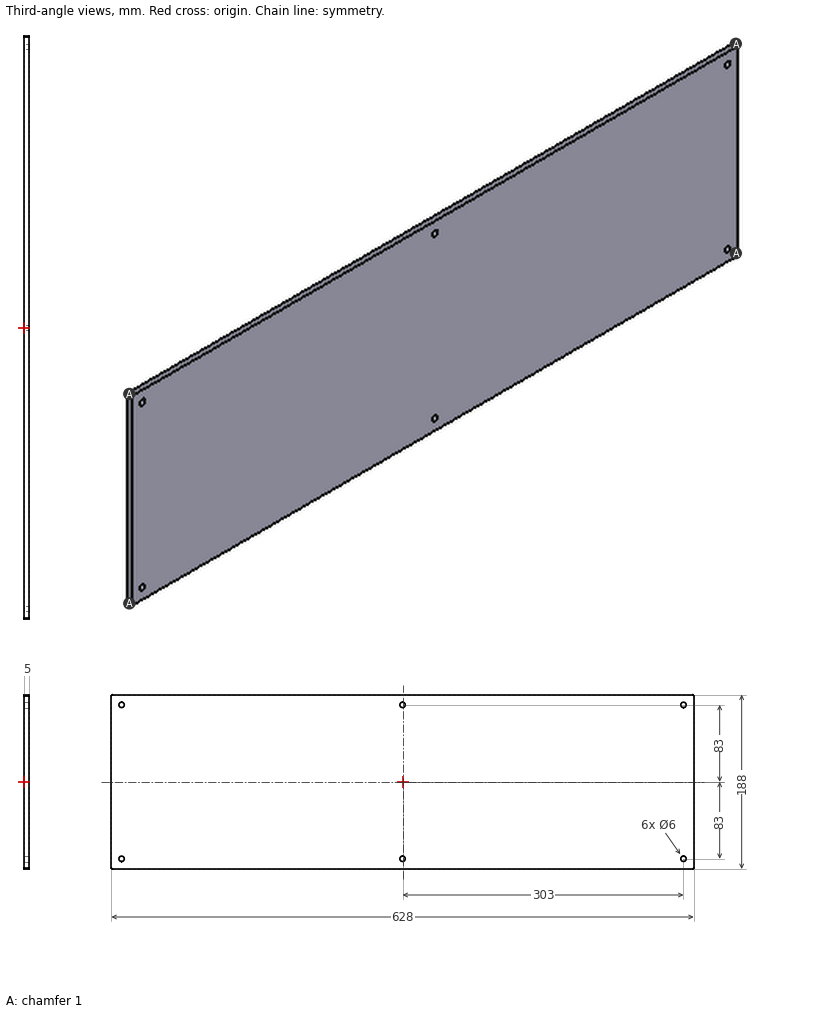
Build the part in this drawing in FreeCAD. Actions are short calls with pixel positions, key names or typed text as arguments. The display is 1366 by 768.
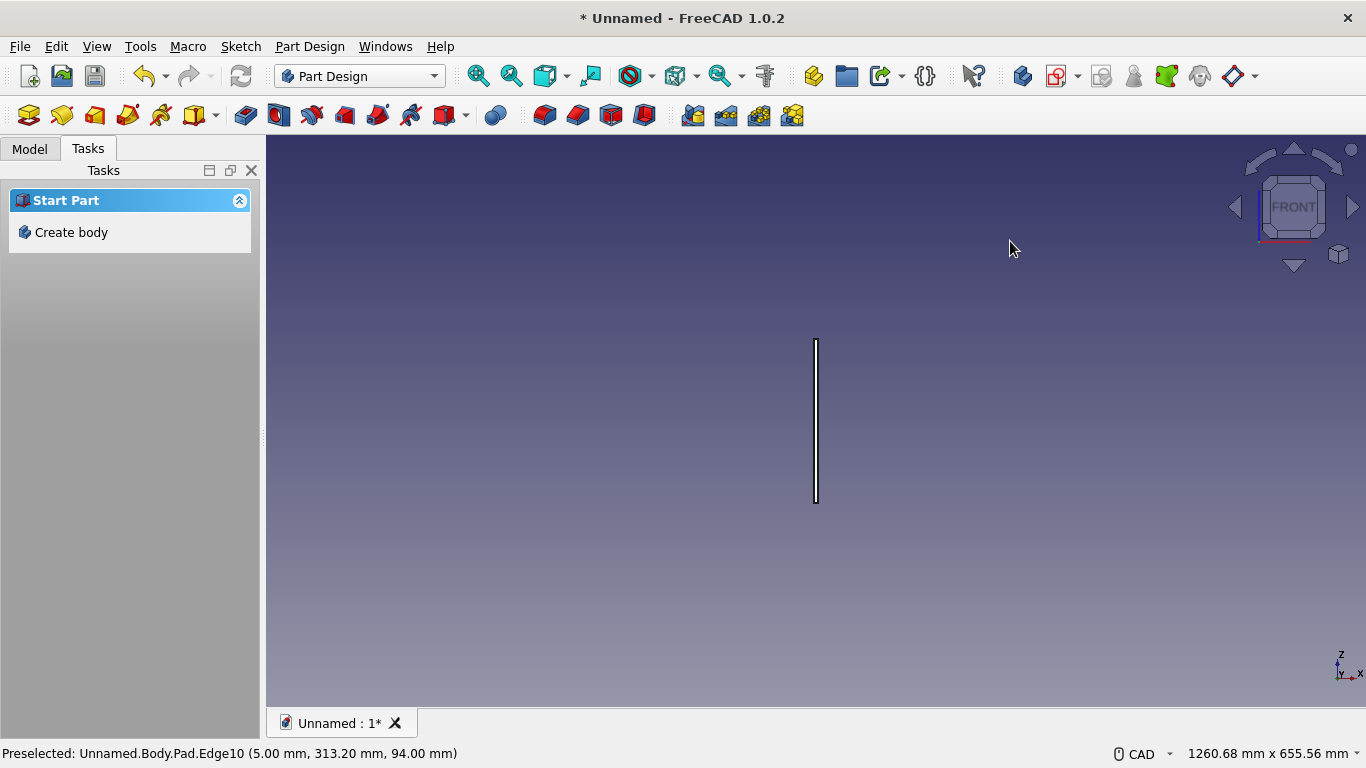
key(v)
key(f)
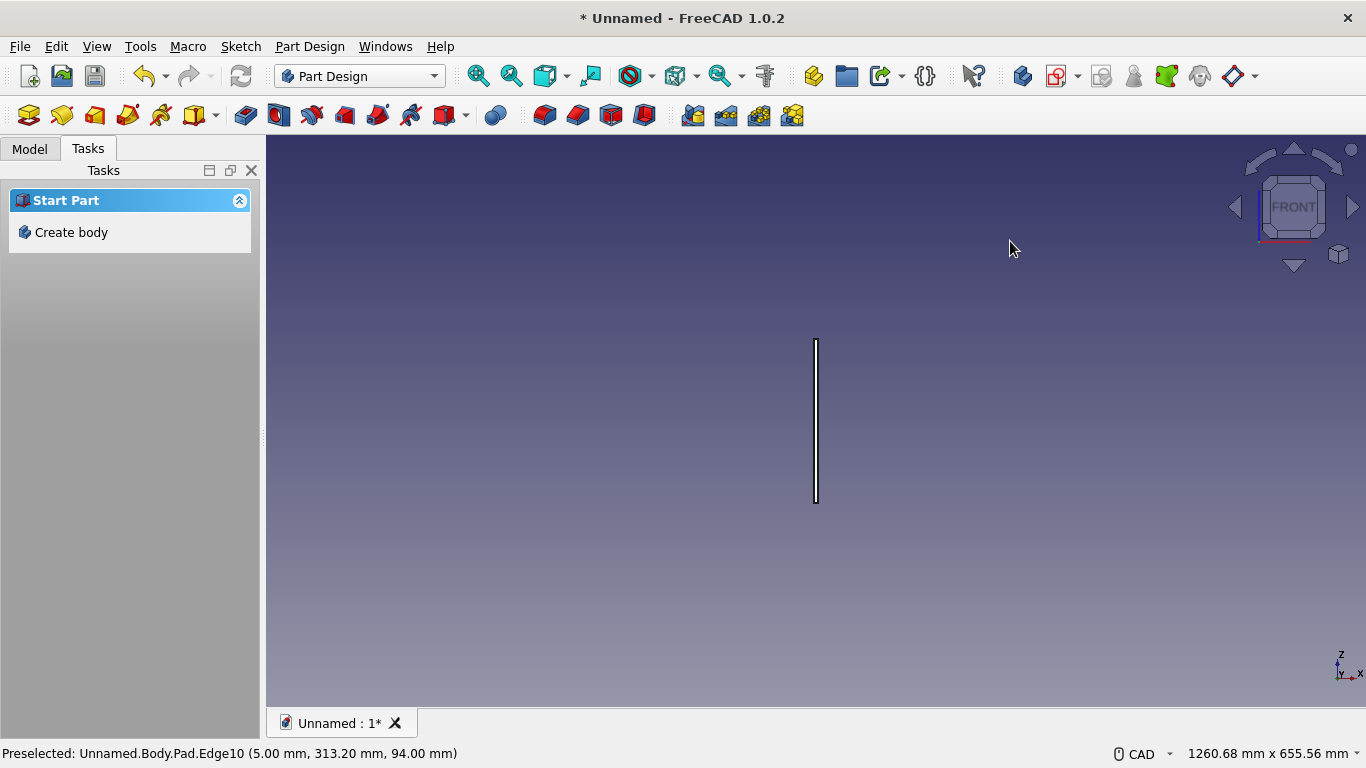
scroll(816, 338, up, 12)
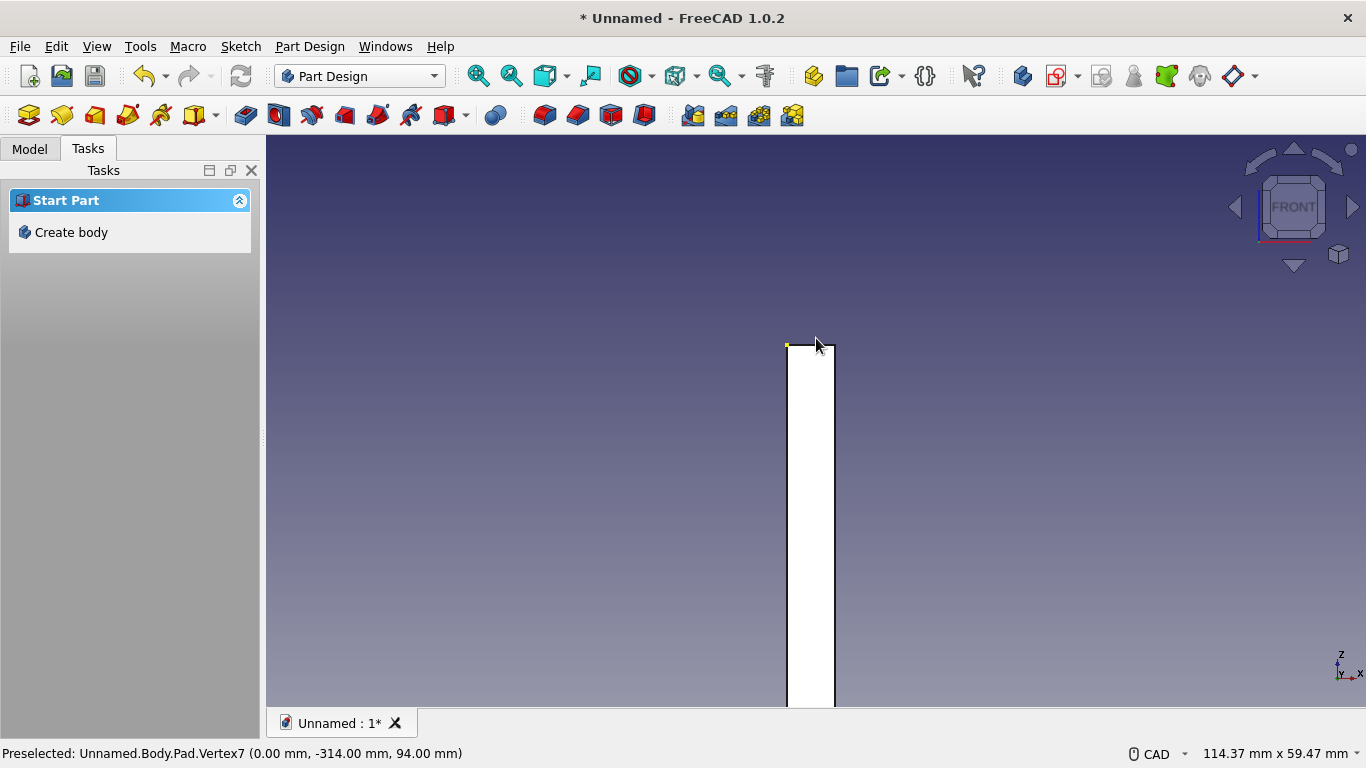
click(811, 344)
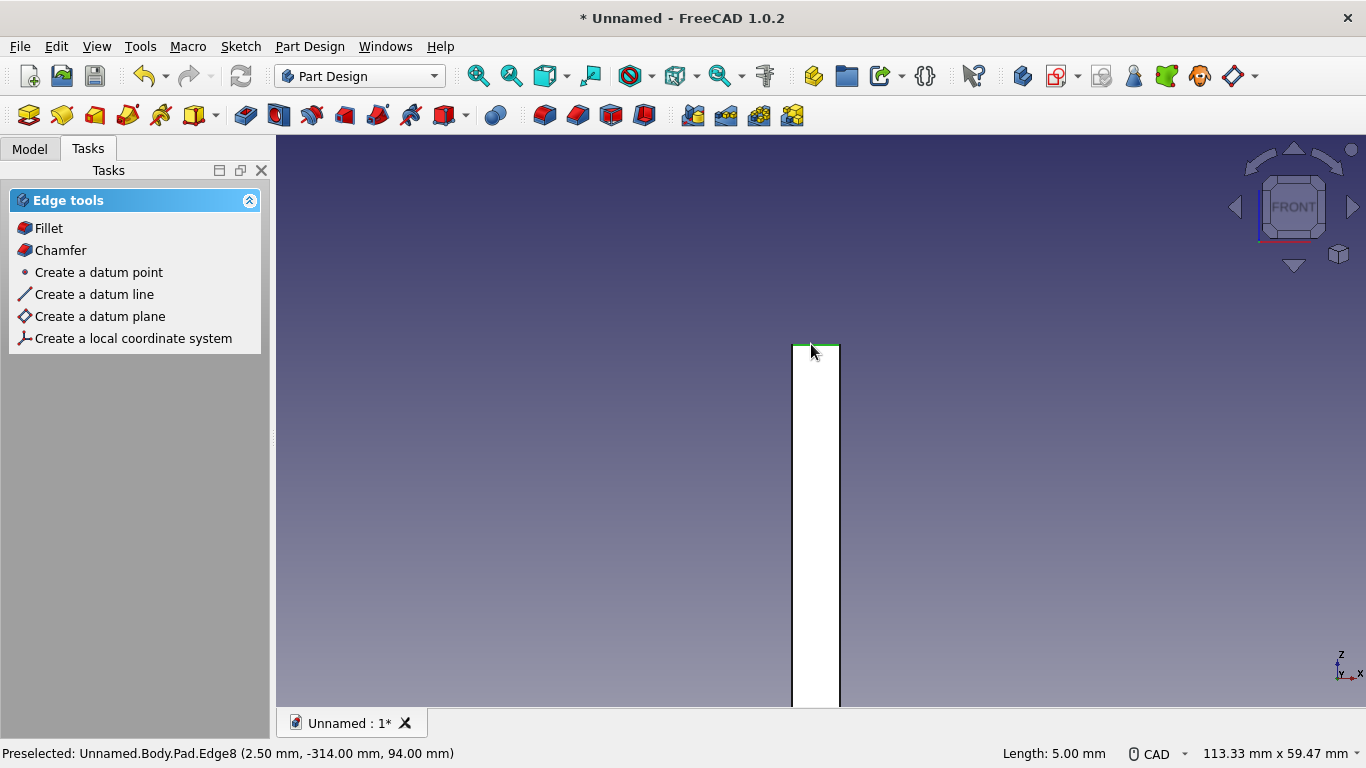
click(479, 76)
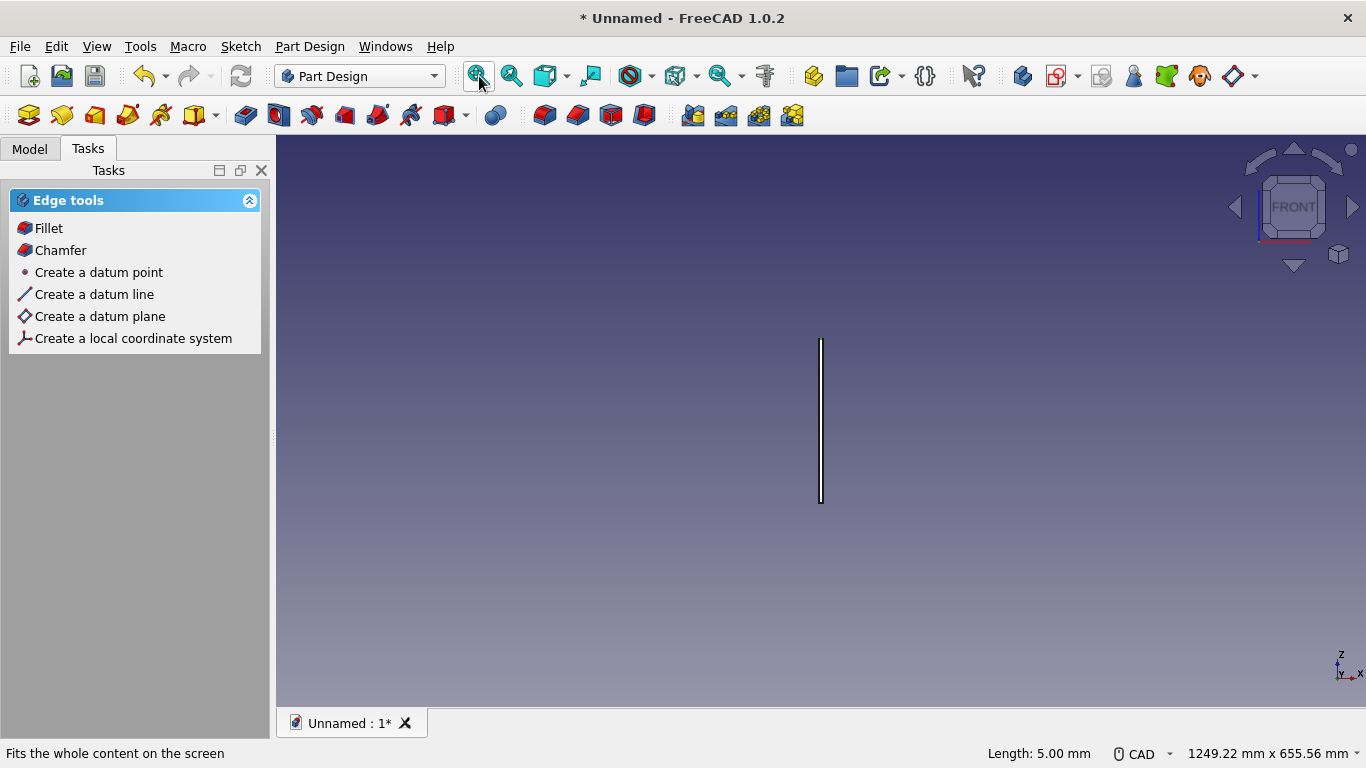
key(3)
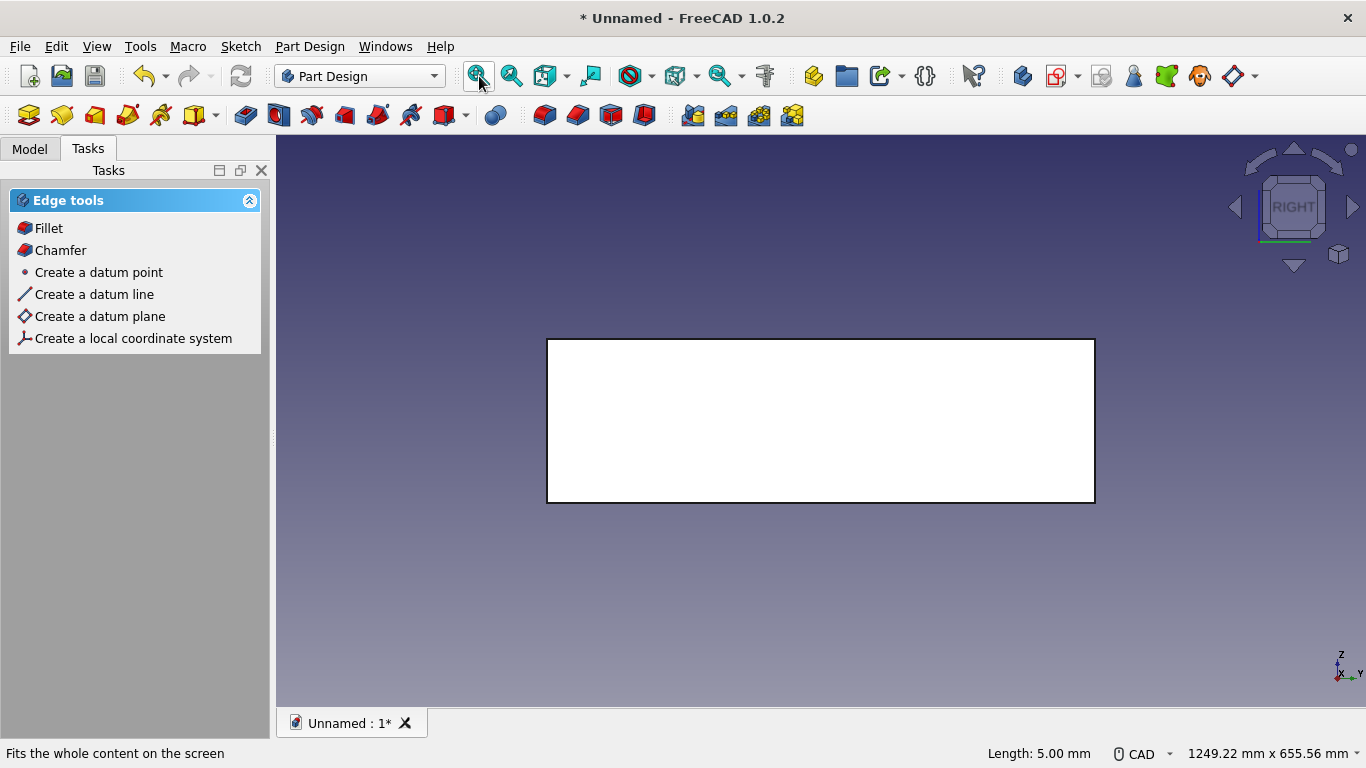
scroll(1095, 338, up, 12)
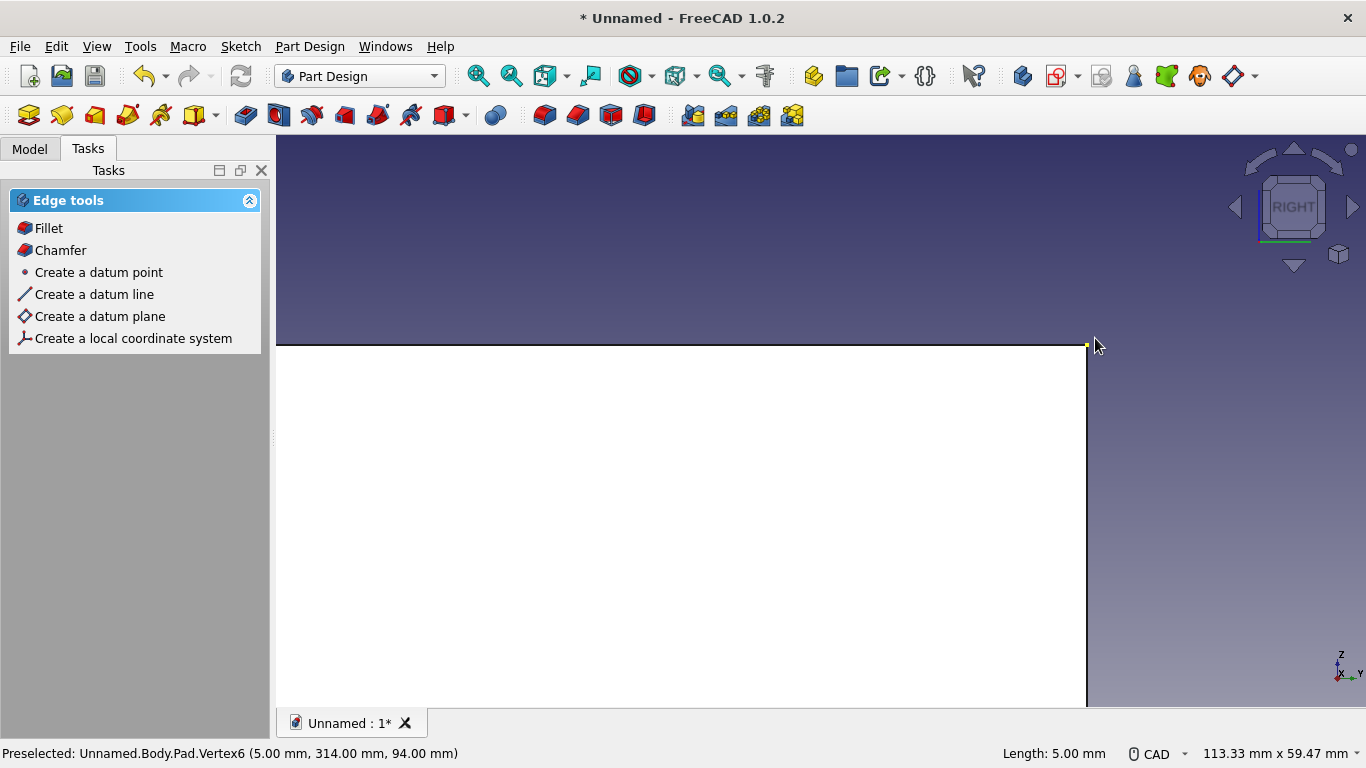
key(v)
key(f)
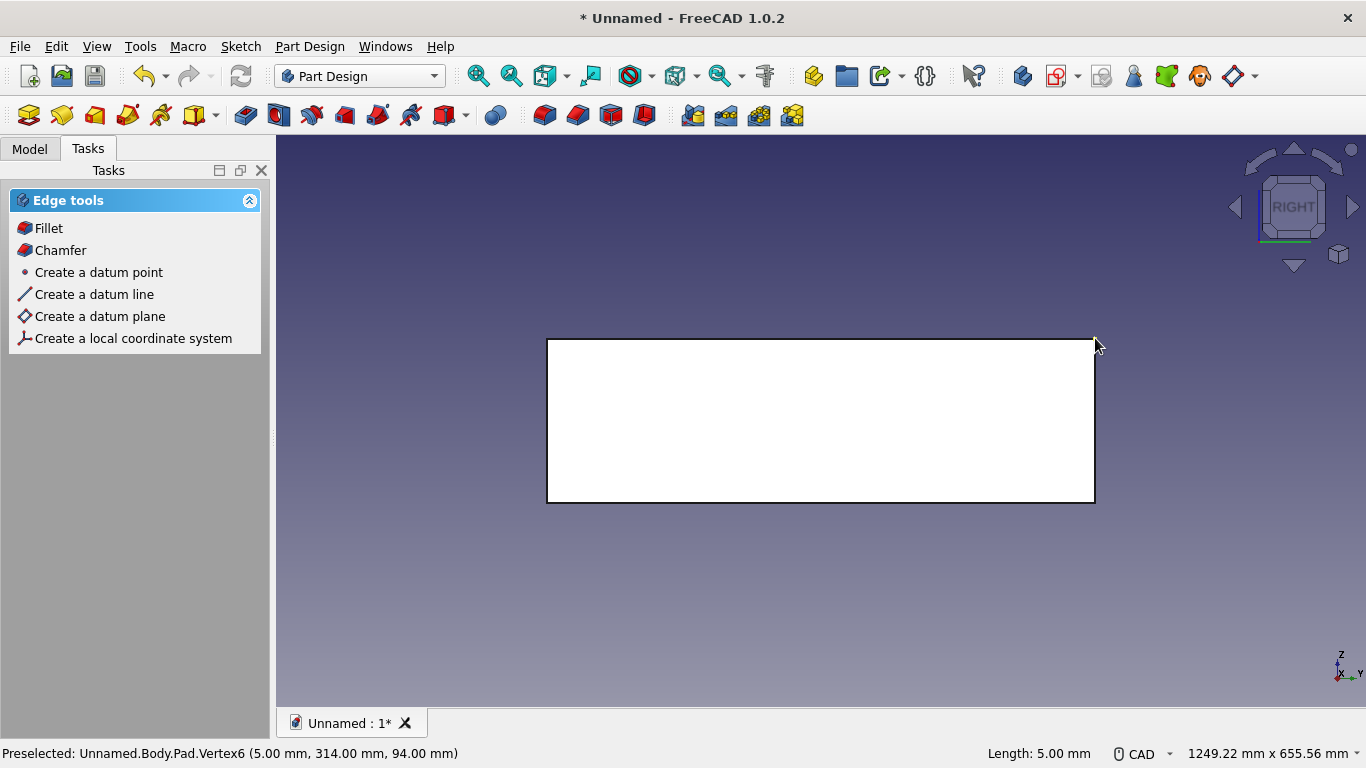
key(5)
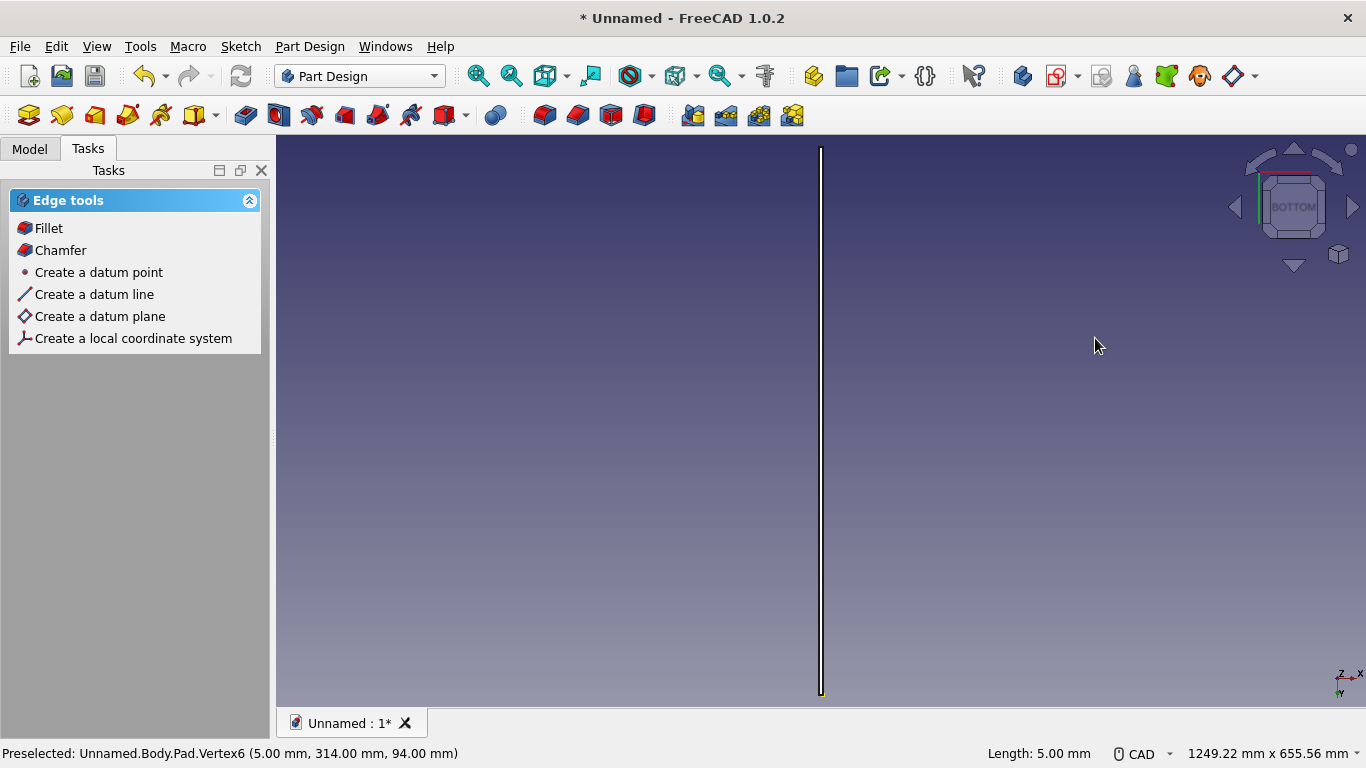
key(4)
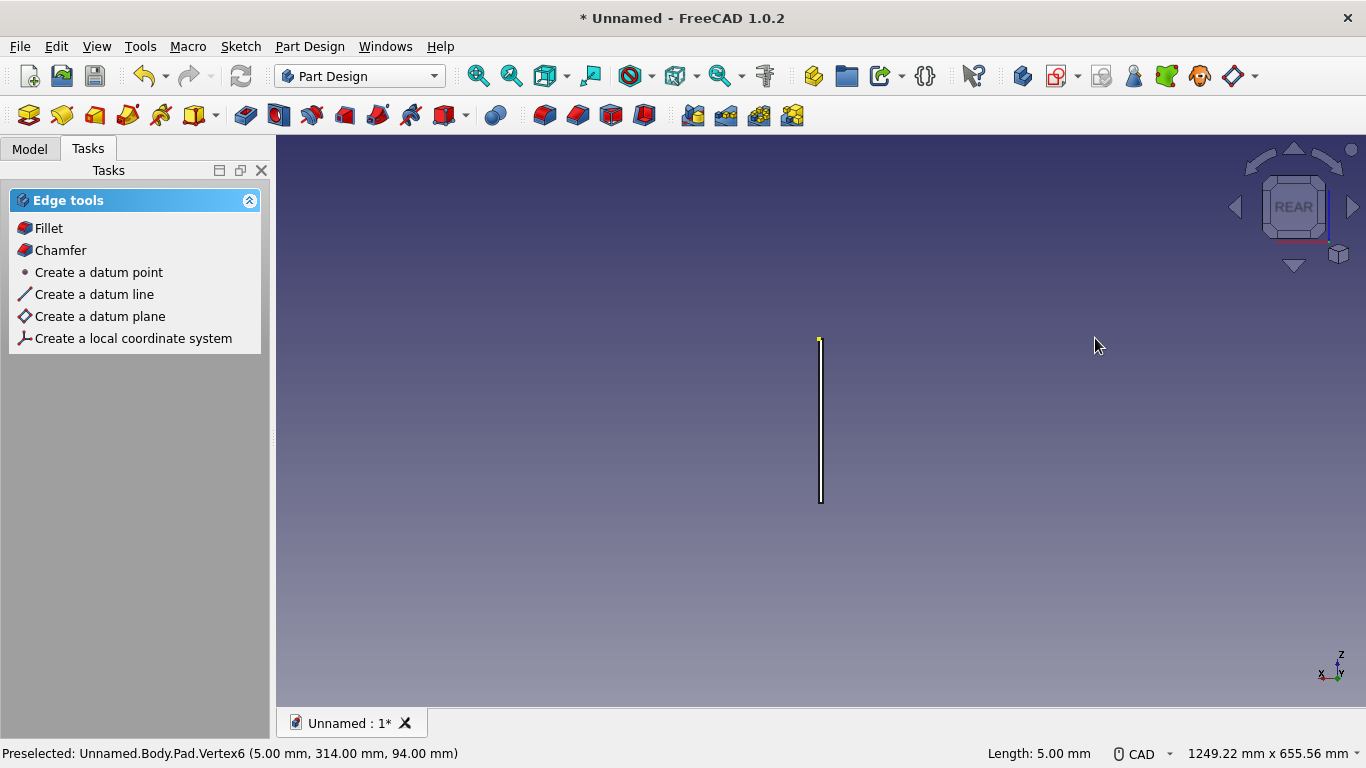
click(479, 76)